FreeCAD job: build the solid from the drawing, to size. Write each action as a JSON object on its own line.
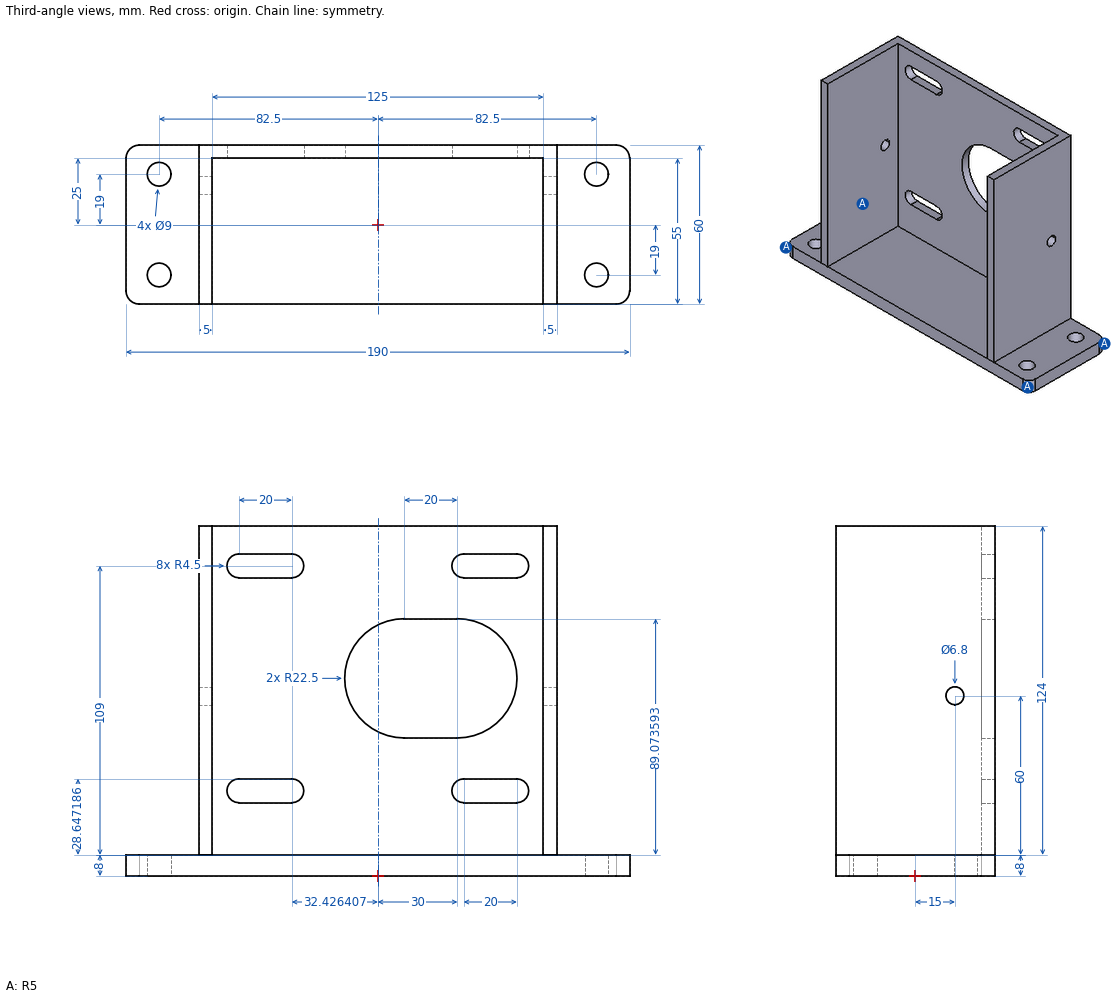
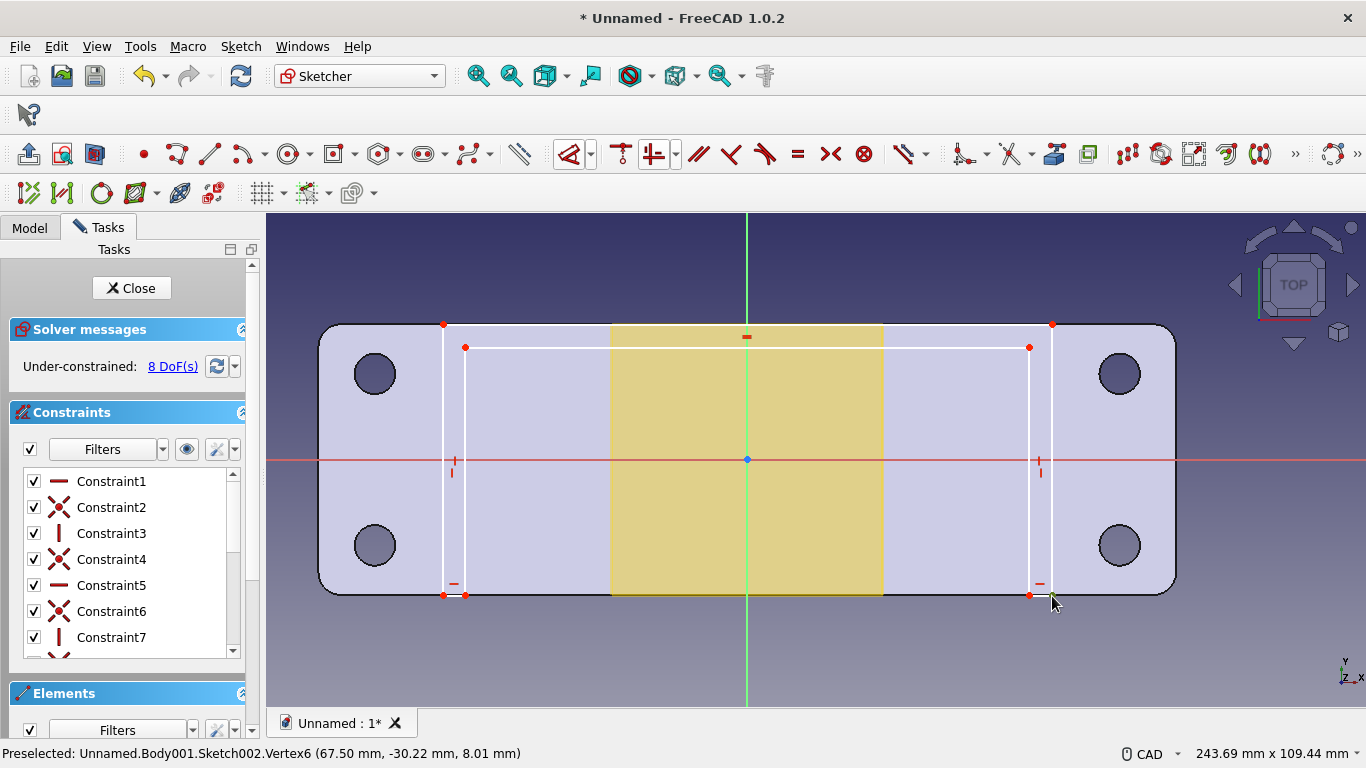
{"action": "left_click", "coordinate": [443, 596]}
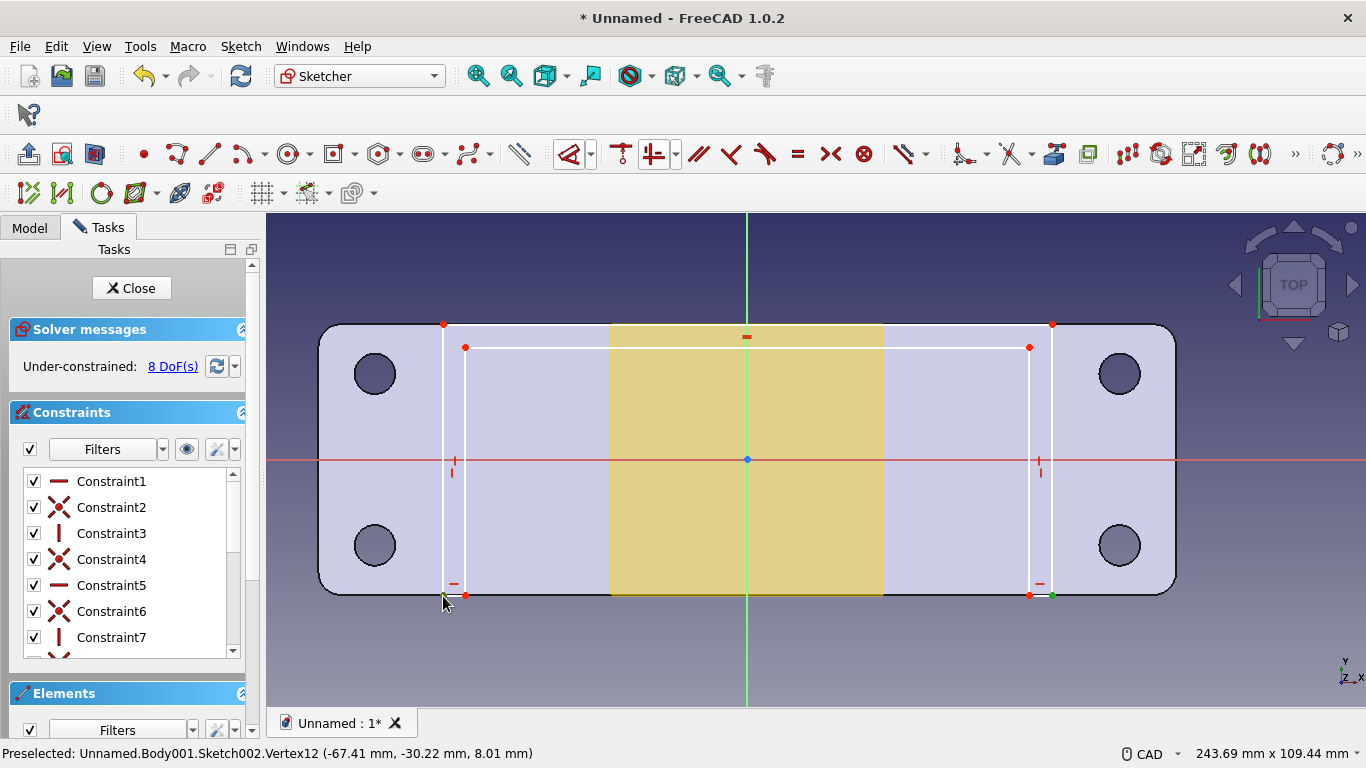
{"action": "left_click", "coordinate": [747, 648]}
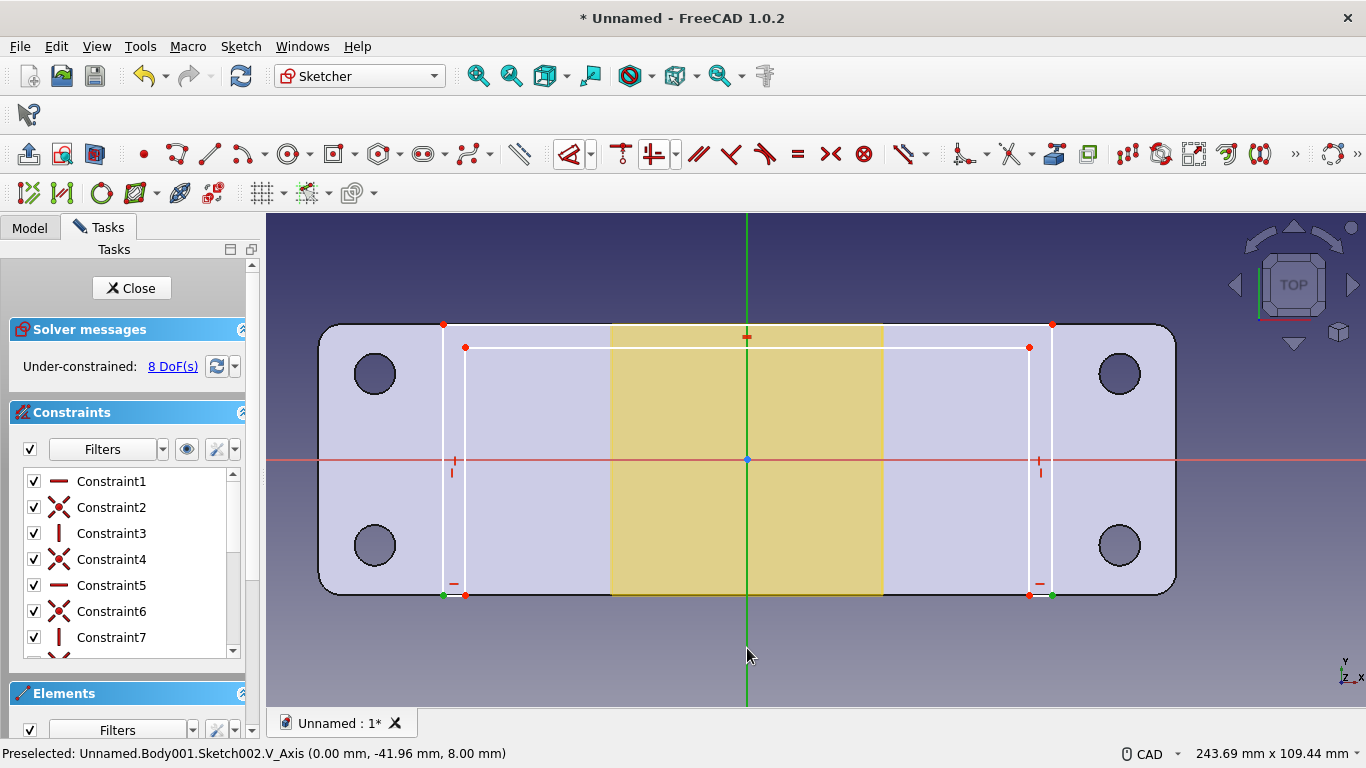
{"action": "left_click", "coordinate": [831, 154]}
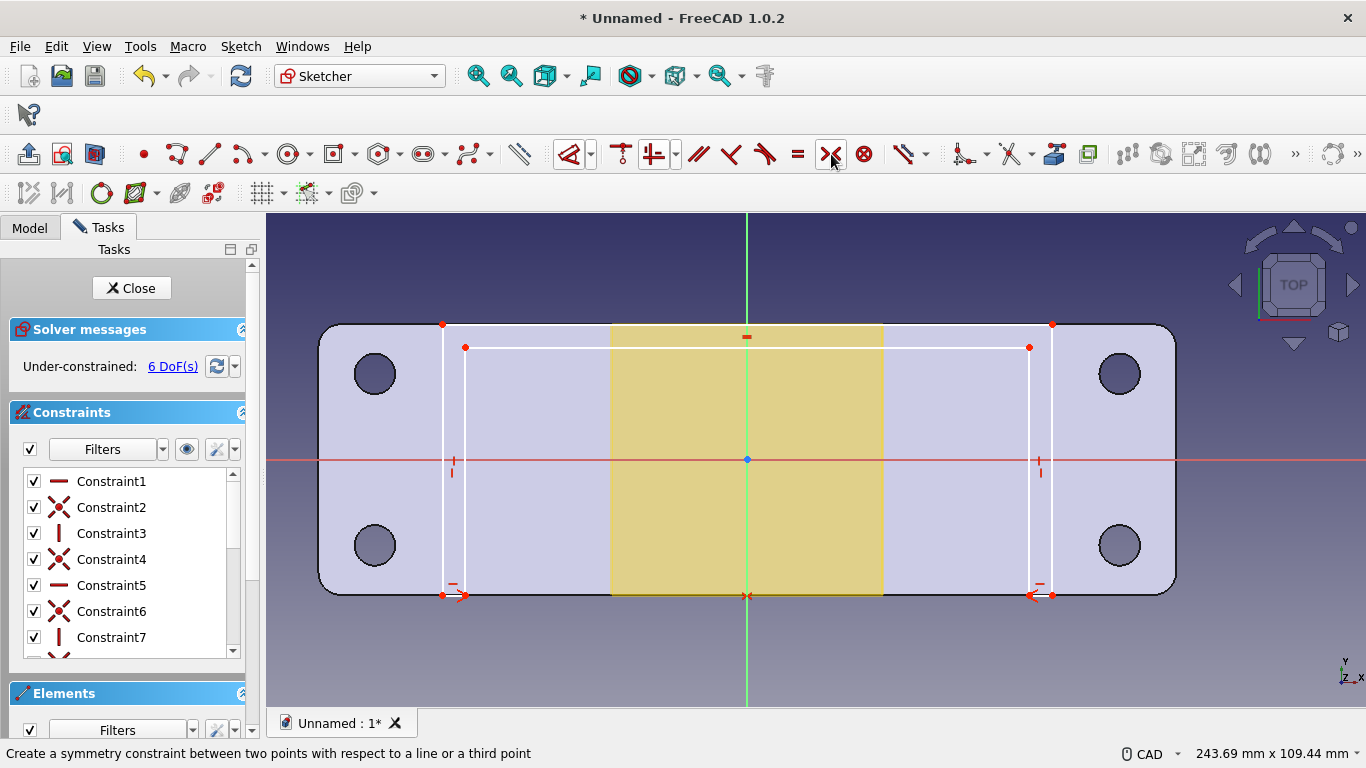
{"action": "left_click", "coordinate": [568, 154]}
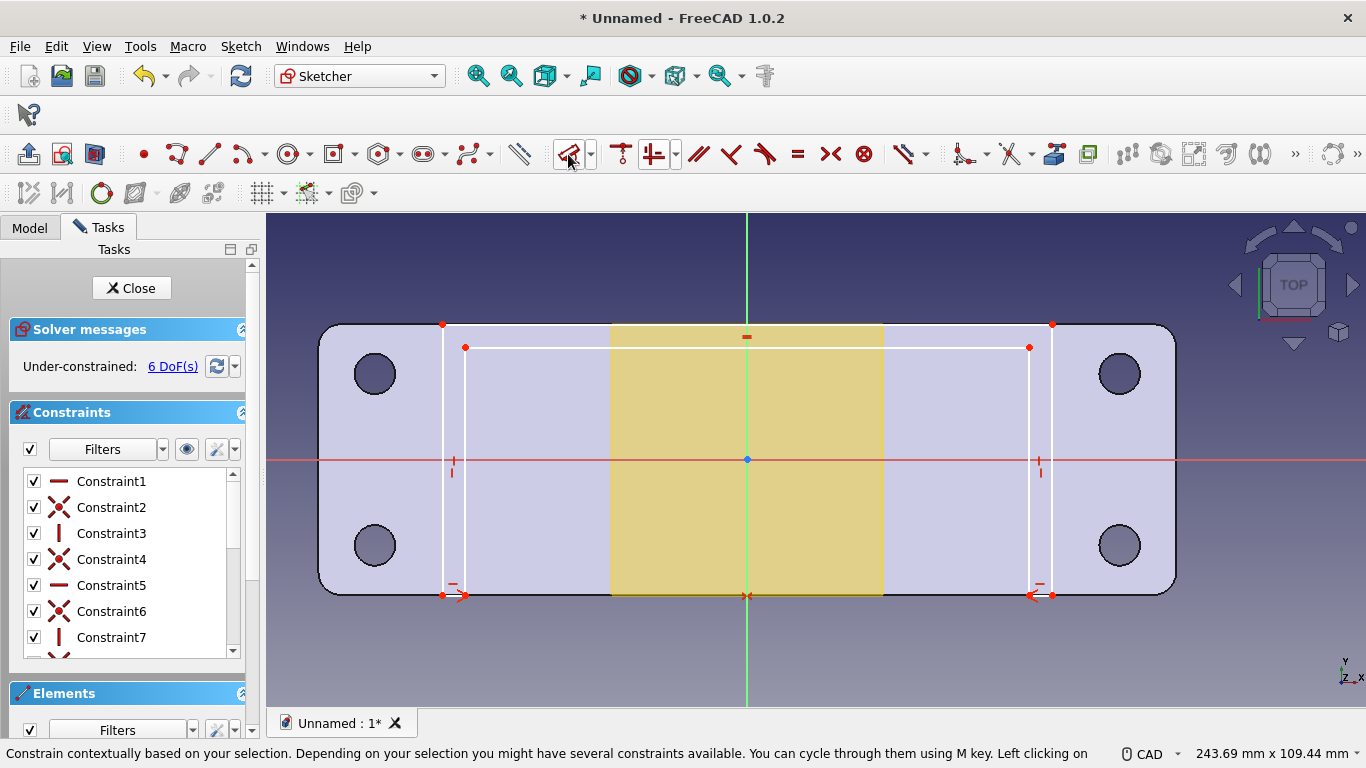
{"action": "scroll", "coordinate": [1038, 596], "scroll_direction": "up", "scroll_amount": 3}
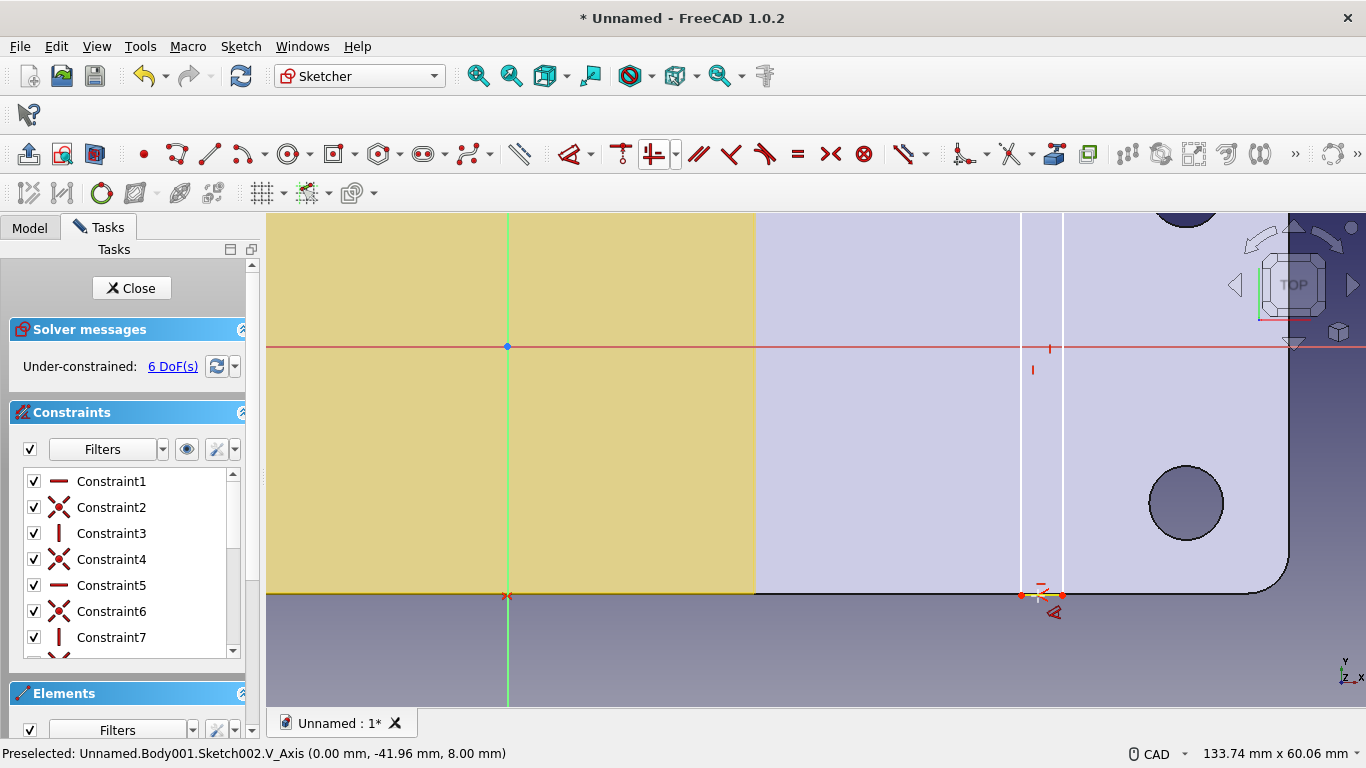
{"action": "left_click", "coordinate": [1038, 595]}
{"action": "left_click", "coordinate": [1042, 629]}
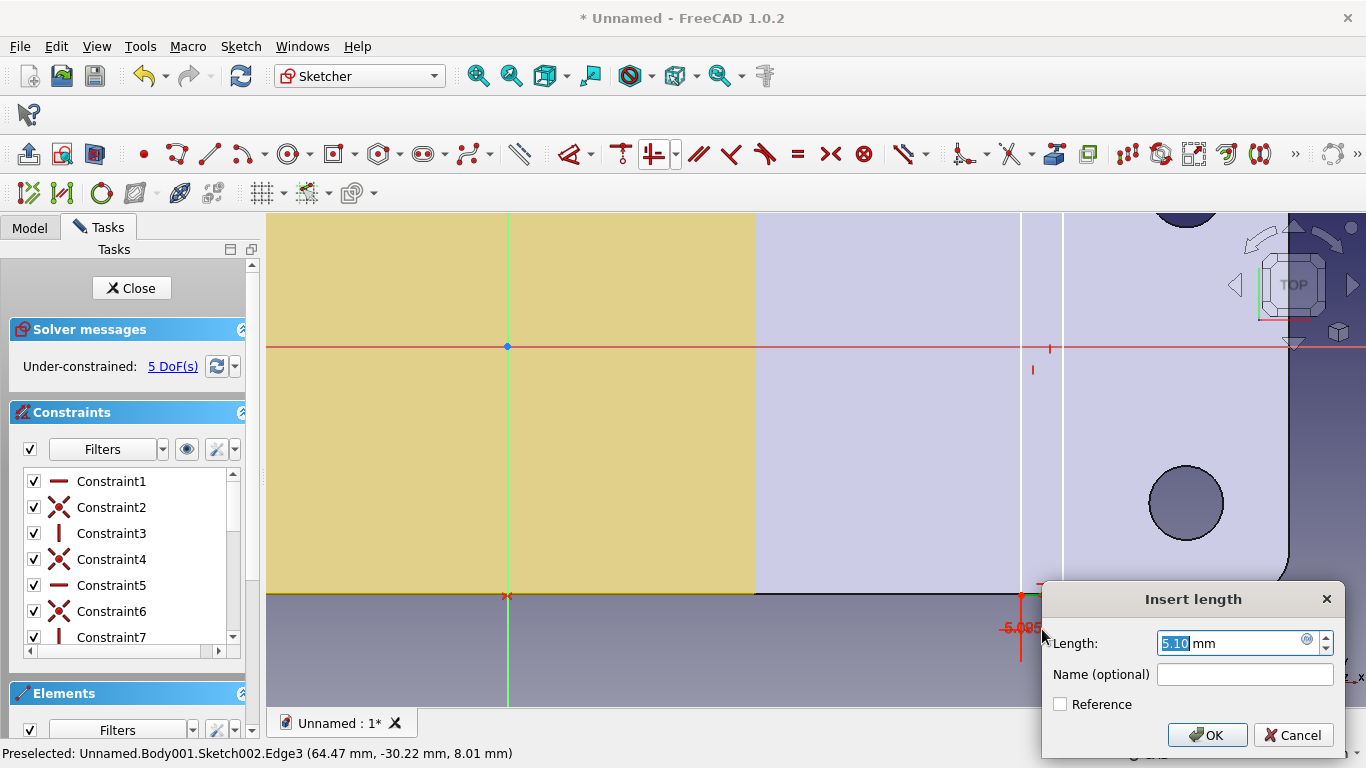
{"action": "type", "text": "5"}
{"action": "key", "text": "Return"}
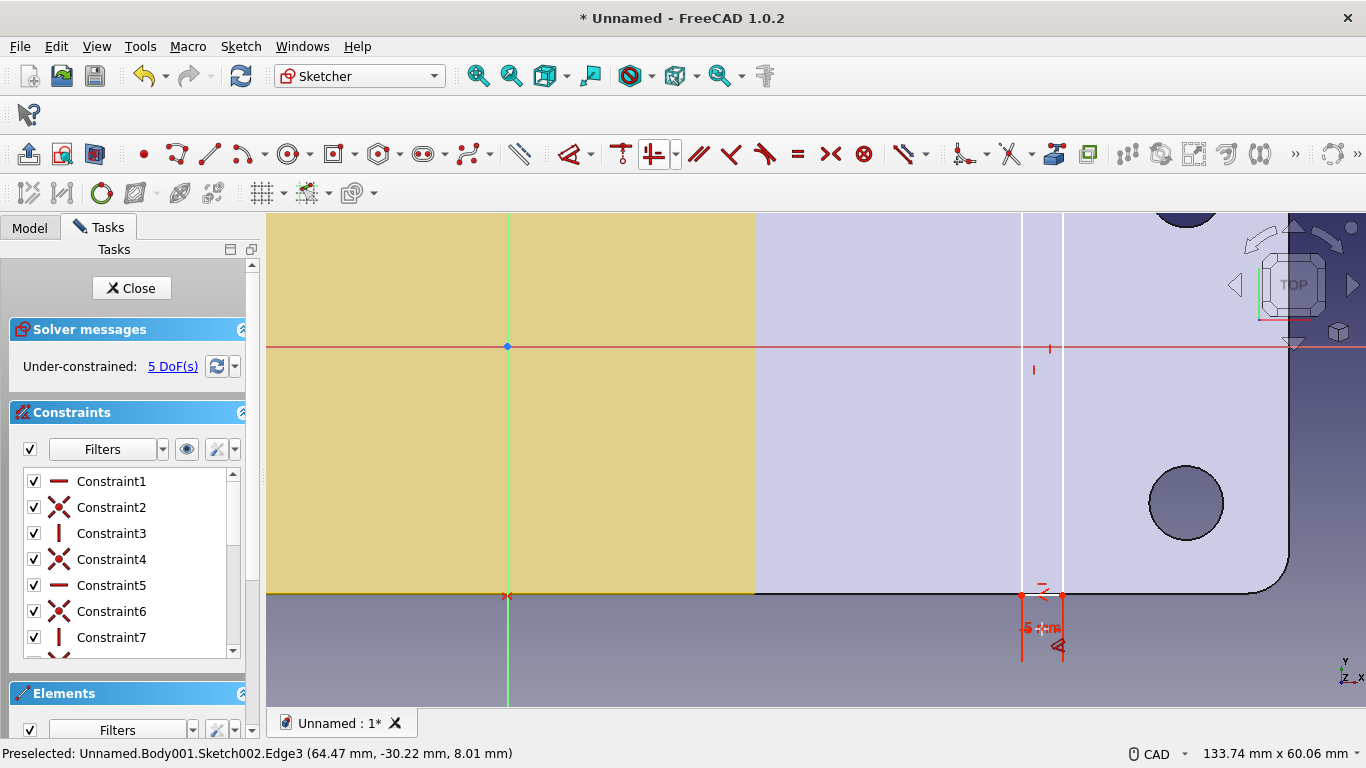
{"action": "scroll", "coordinate": [1039, 598], "scroll_direction": "down", "scroll_amount": 3}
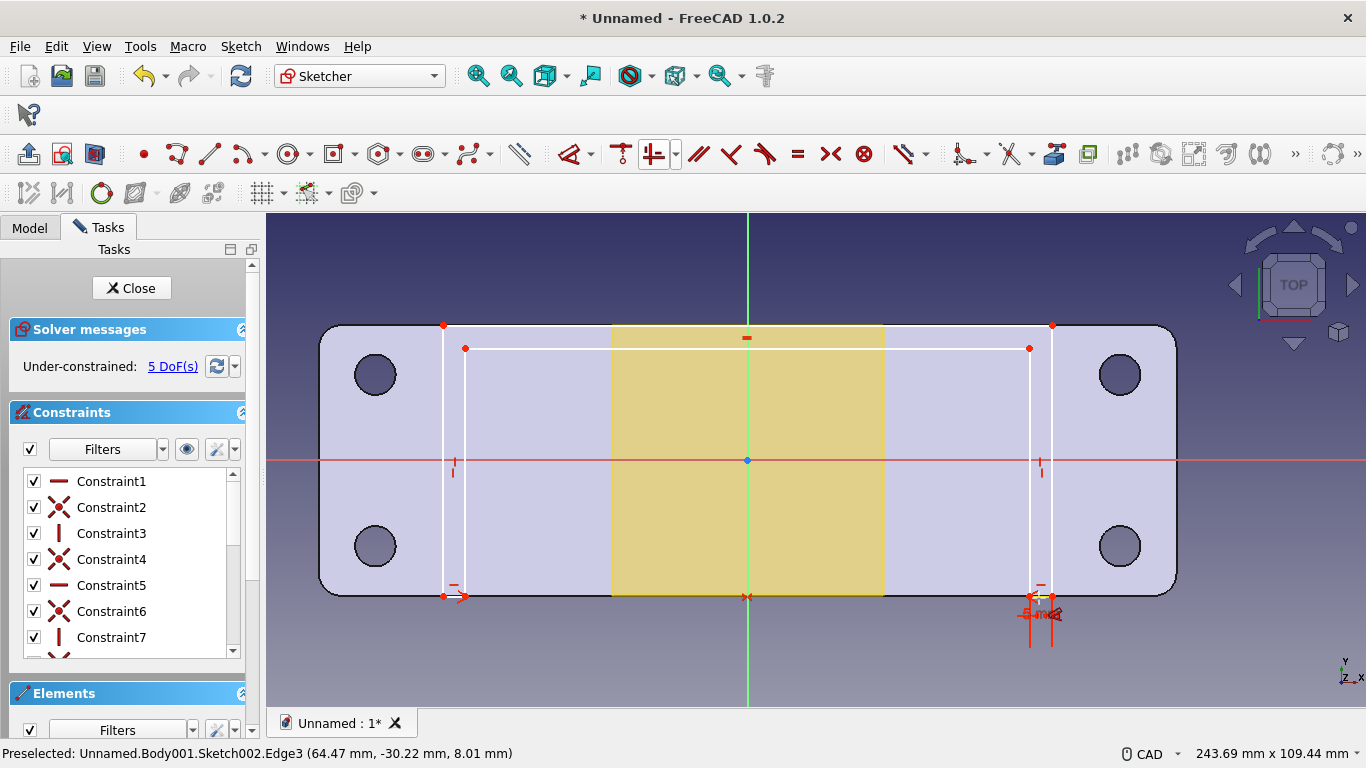
{"action": "scroll", "coordinate": [450, 597], "scroll_direction": "up", "scroll_amount": 4}